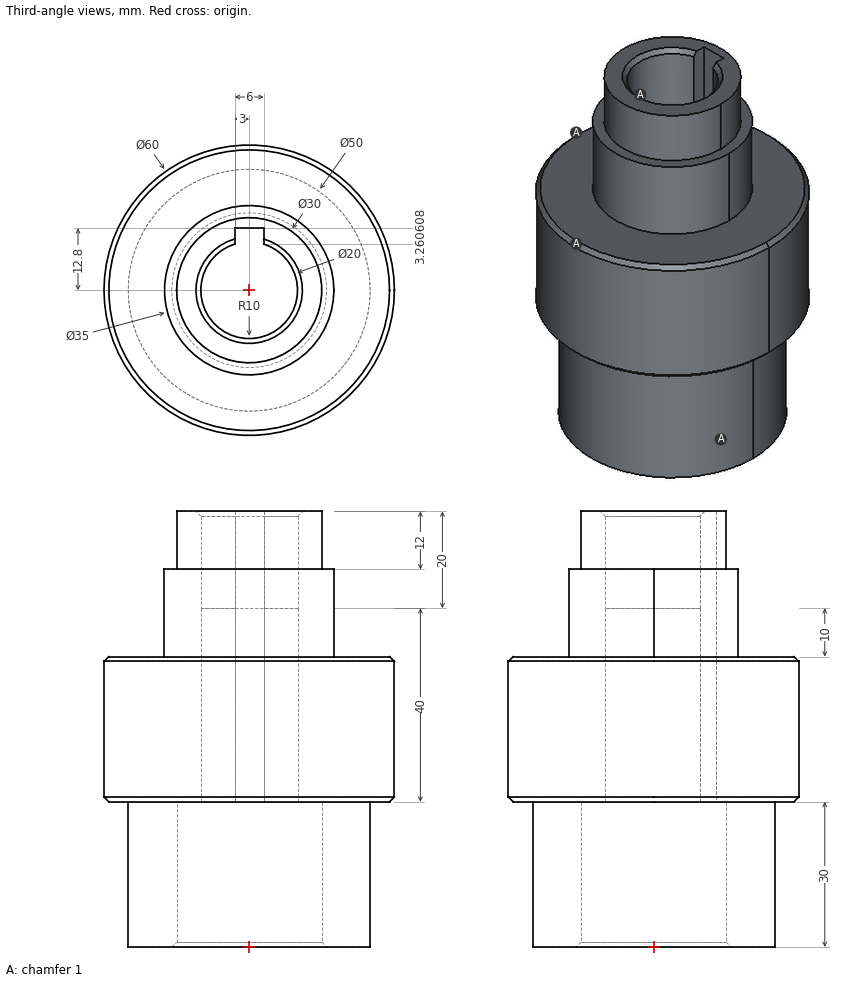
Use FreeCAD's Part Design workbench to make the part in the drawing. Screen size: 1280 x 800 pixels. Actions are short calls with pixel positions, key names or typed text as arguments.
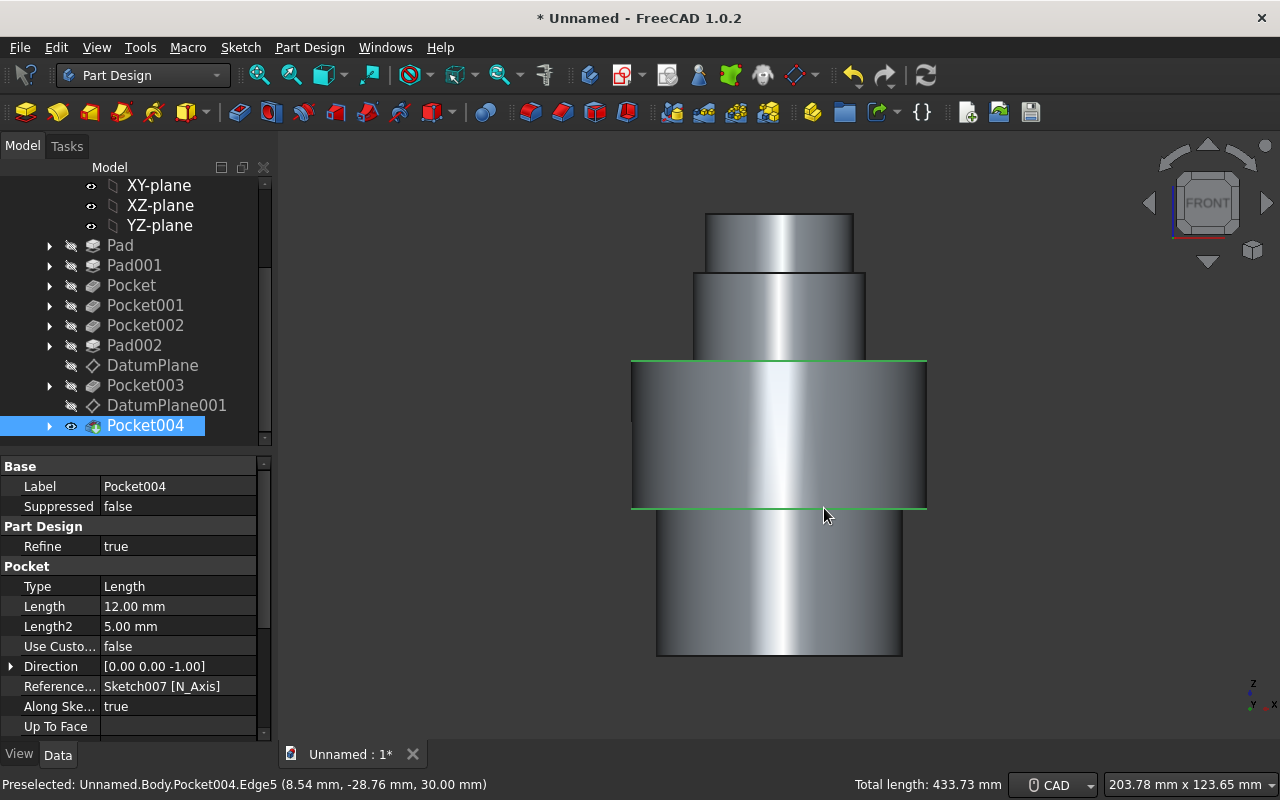
key(3)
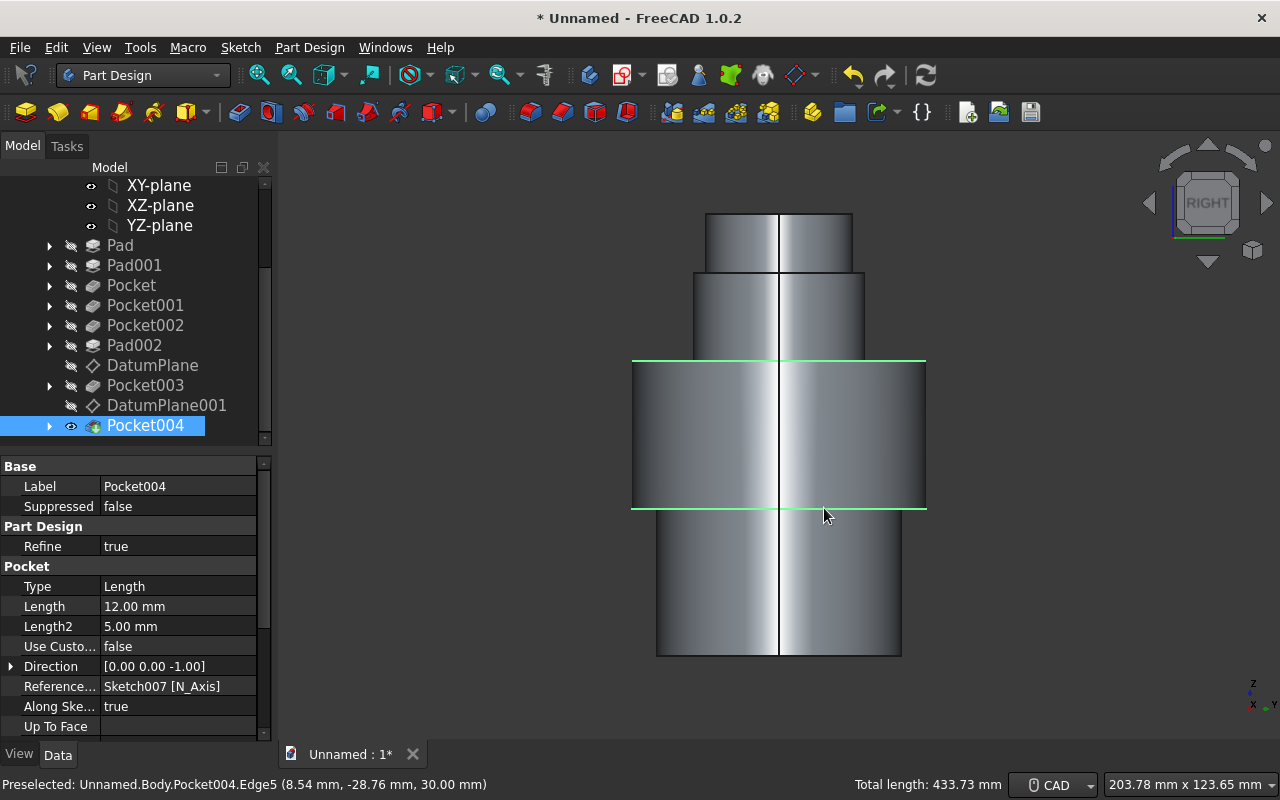
key(5)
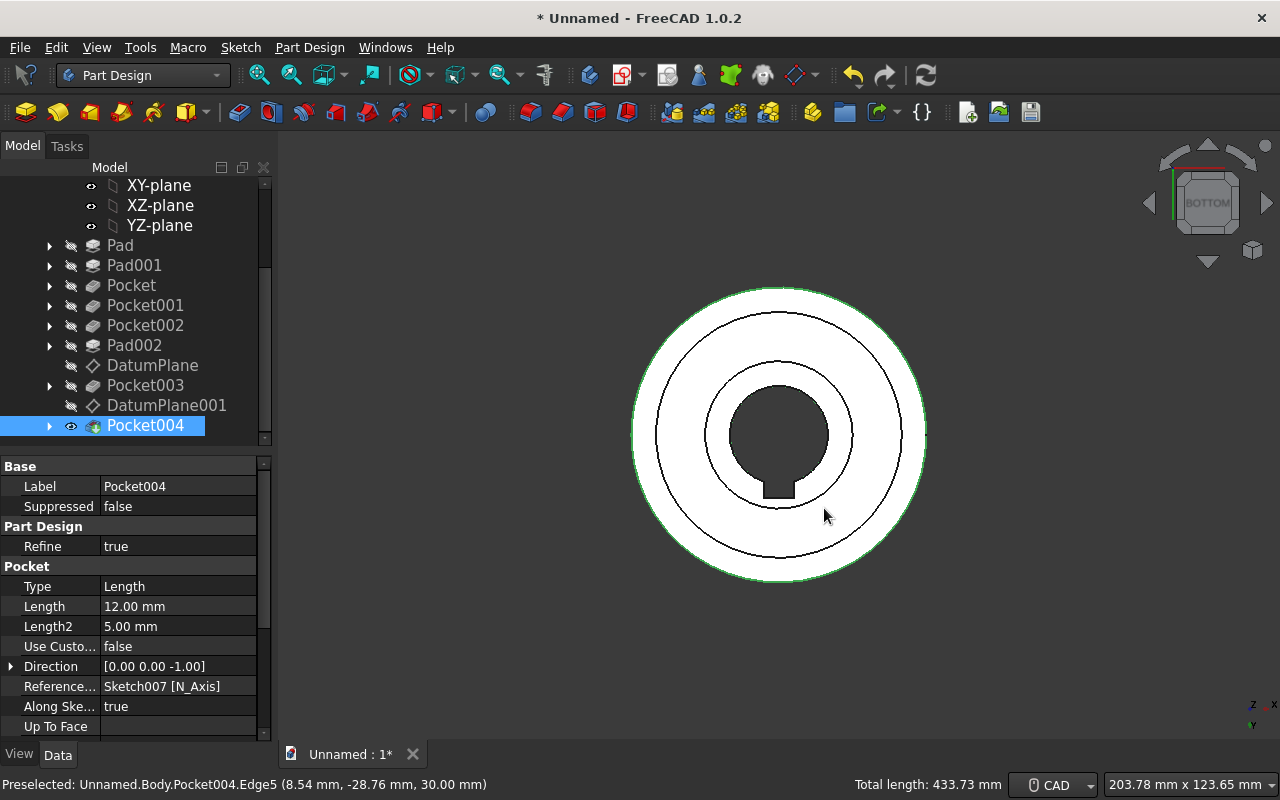
click(705, 434, ctrl)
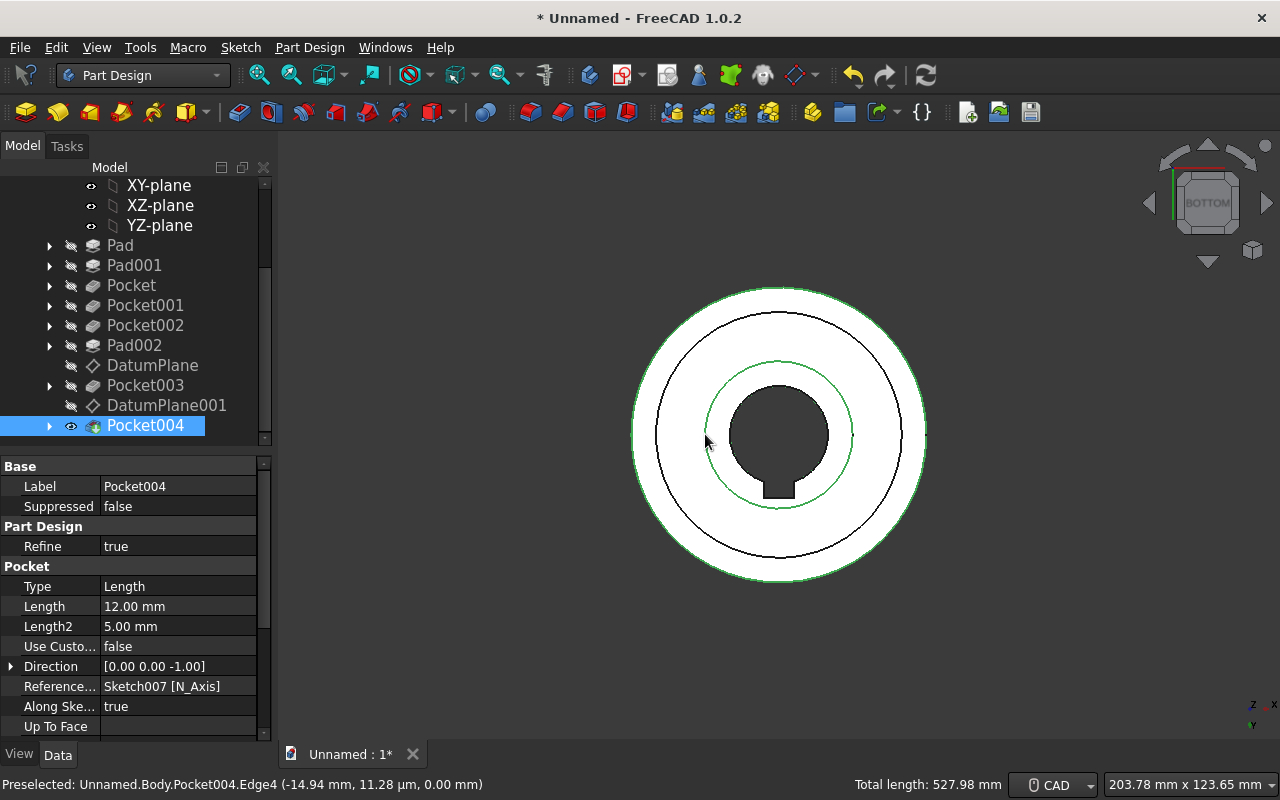
click(564, 112)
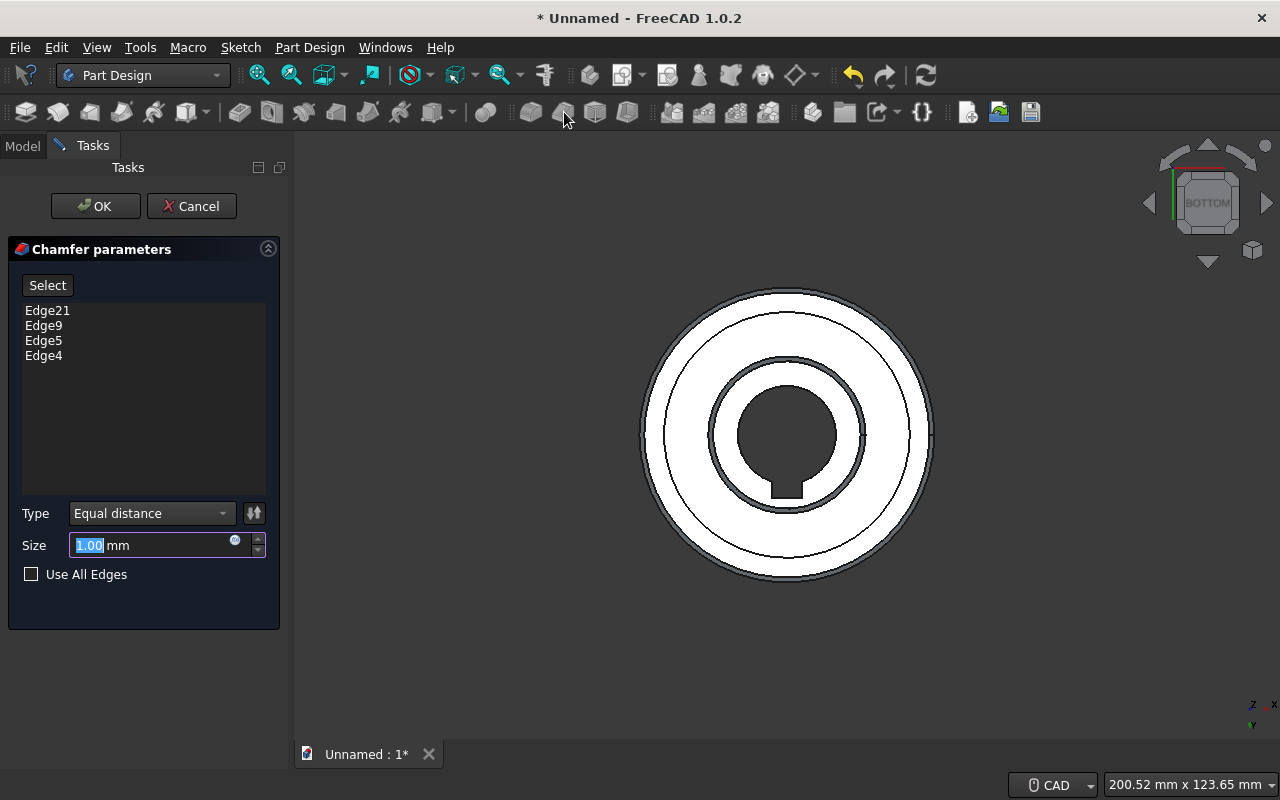
text(1)
key(Tab)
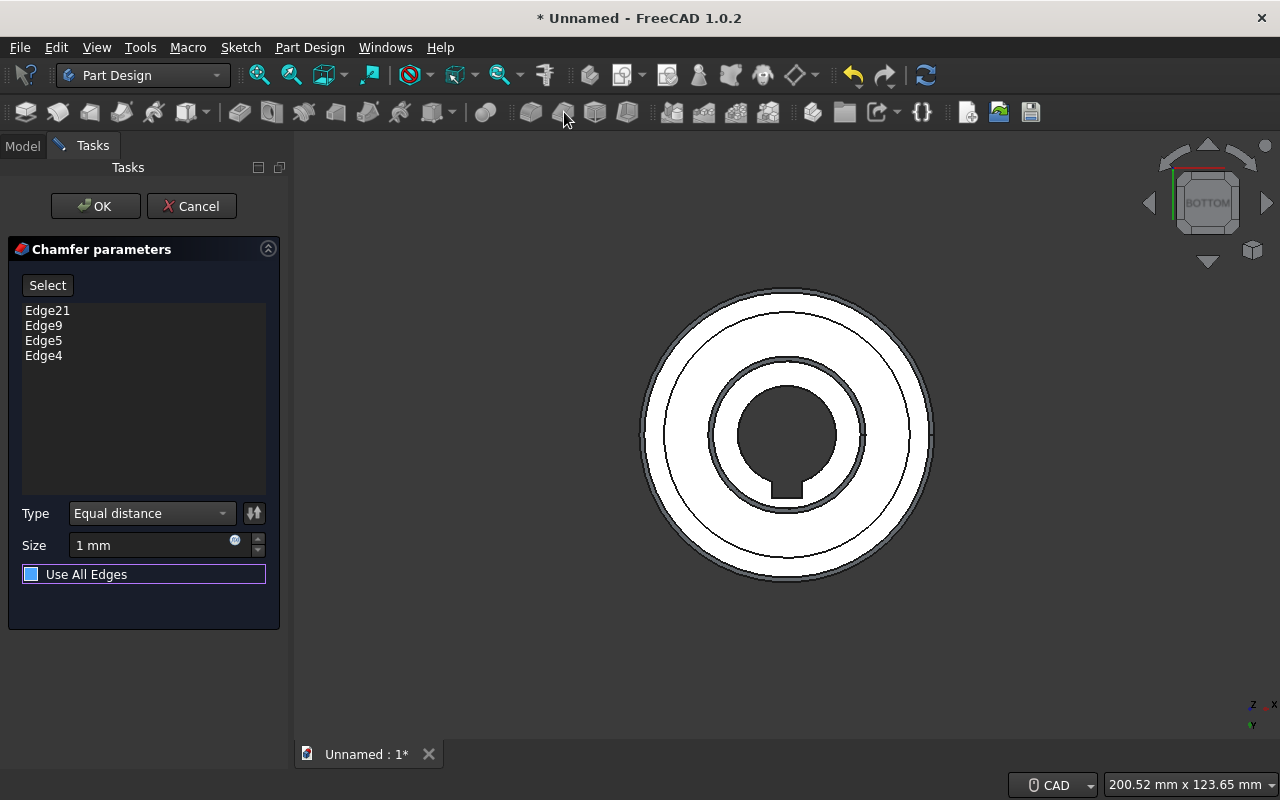
click(96, 206)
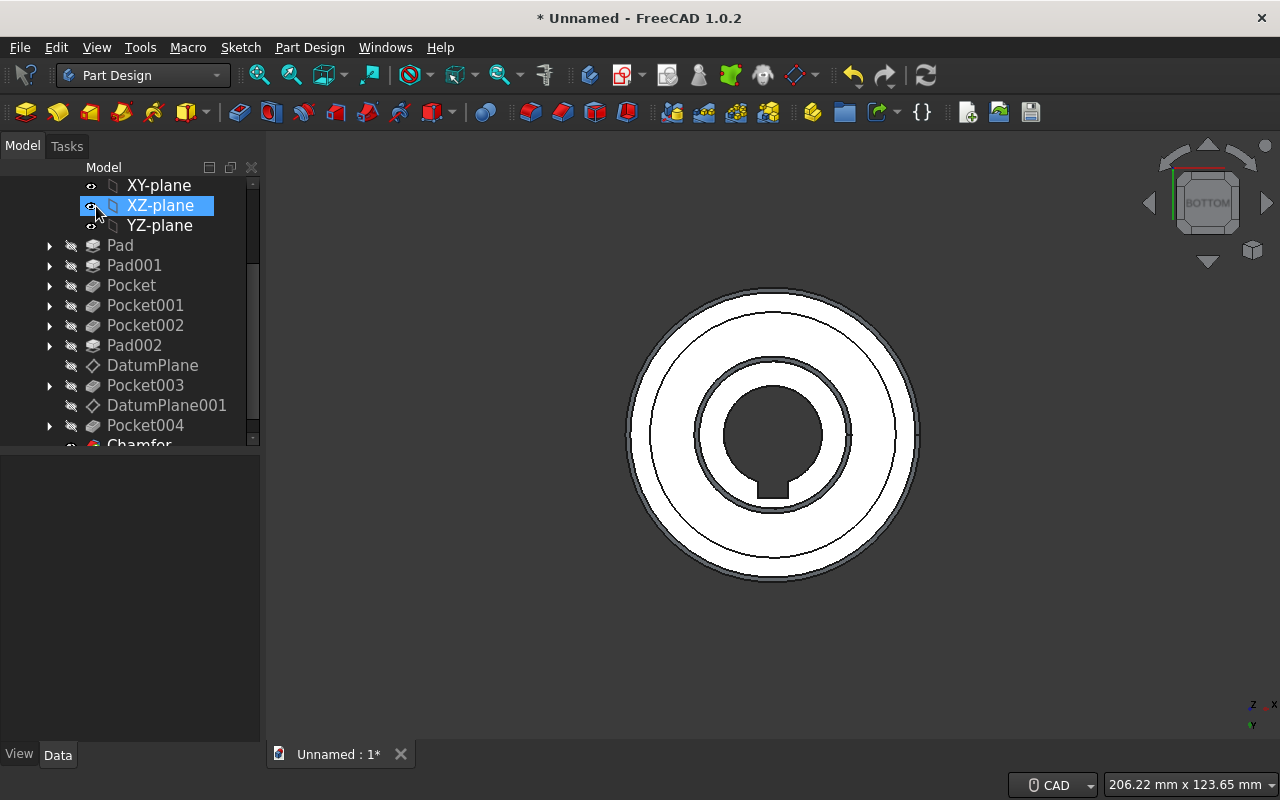
key(0)